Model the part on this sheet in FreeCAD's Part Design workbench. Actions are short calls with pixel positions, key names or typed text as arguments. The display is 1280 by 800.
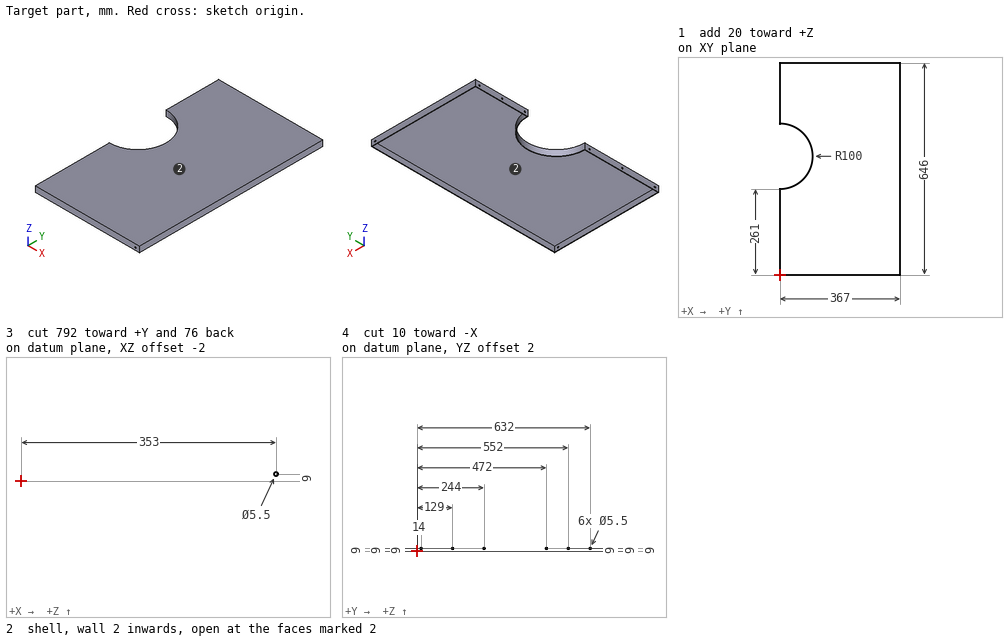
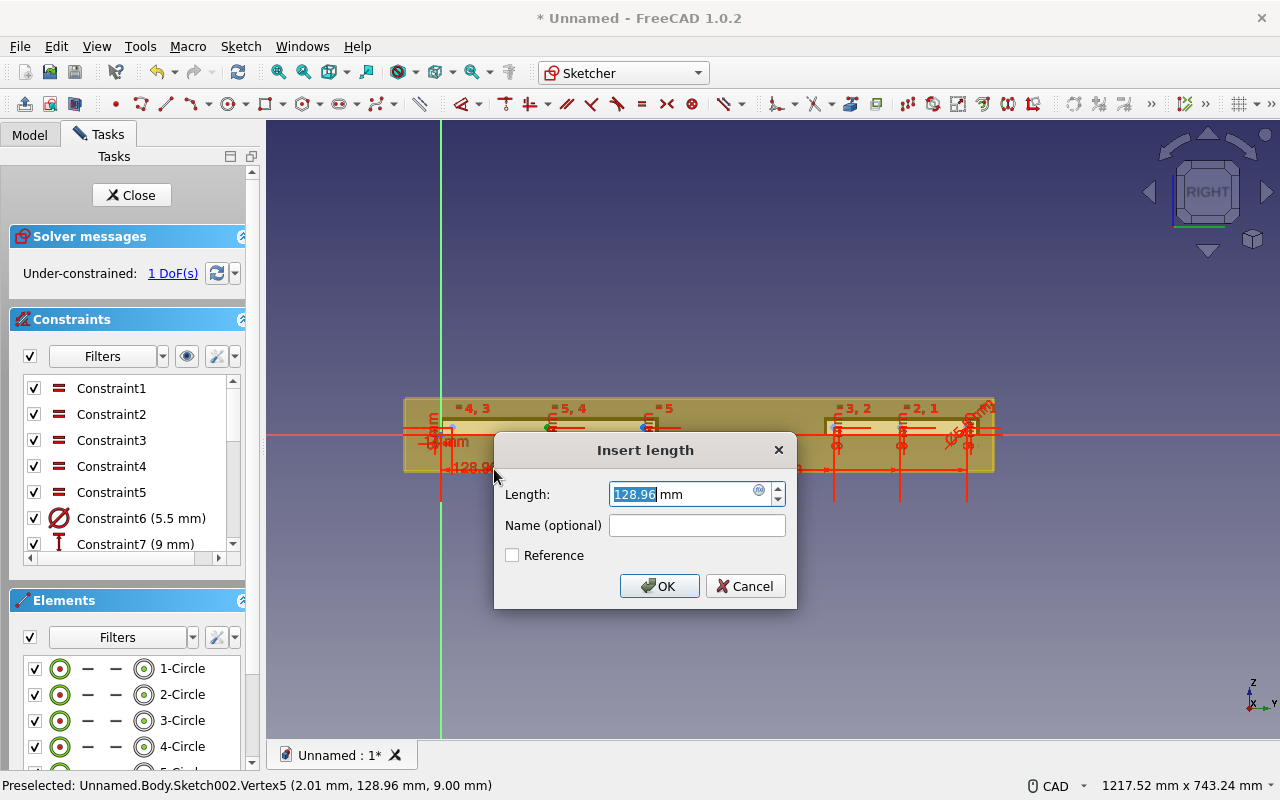
text(129)
key(Return)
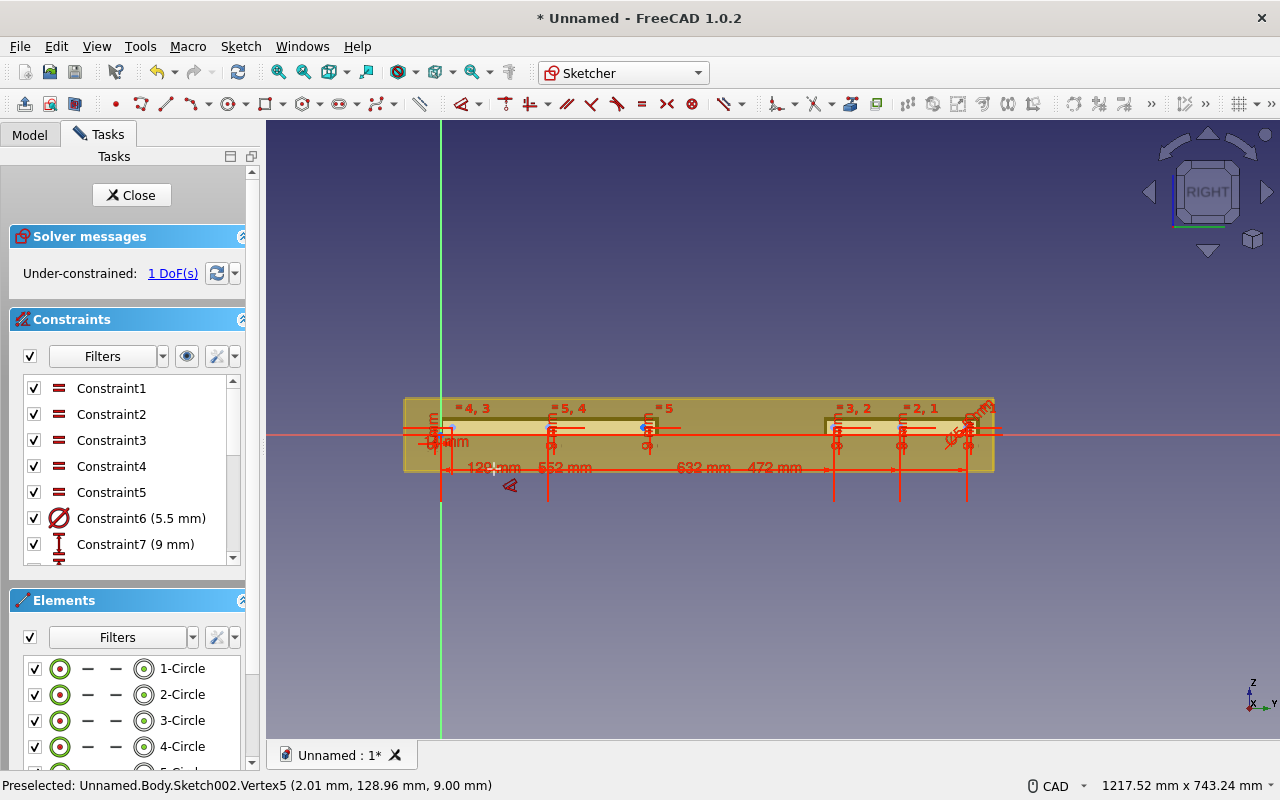
click(644, 428)
click(542, 394)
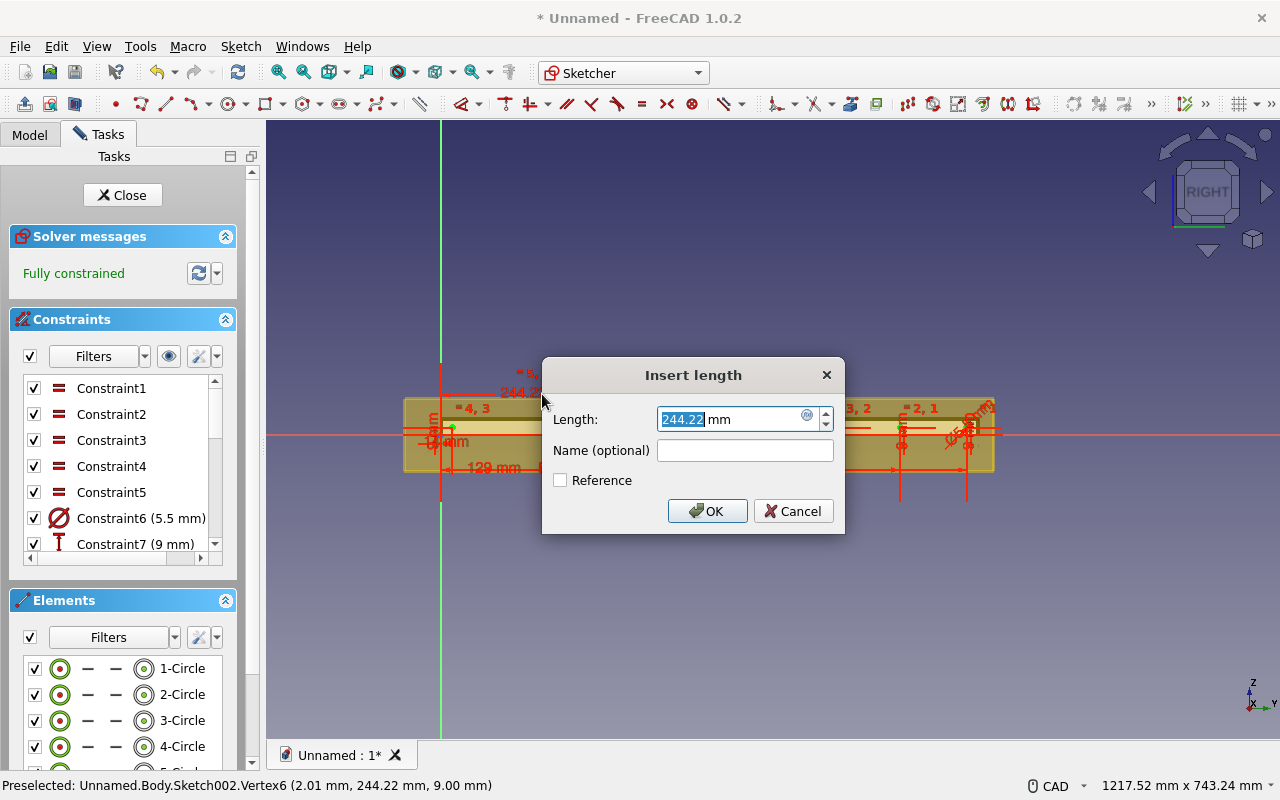
text(244)
key(Return)
key(Escape)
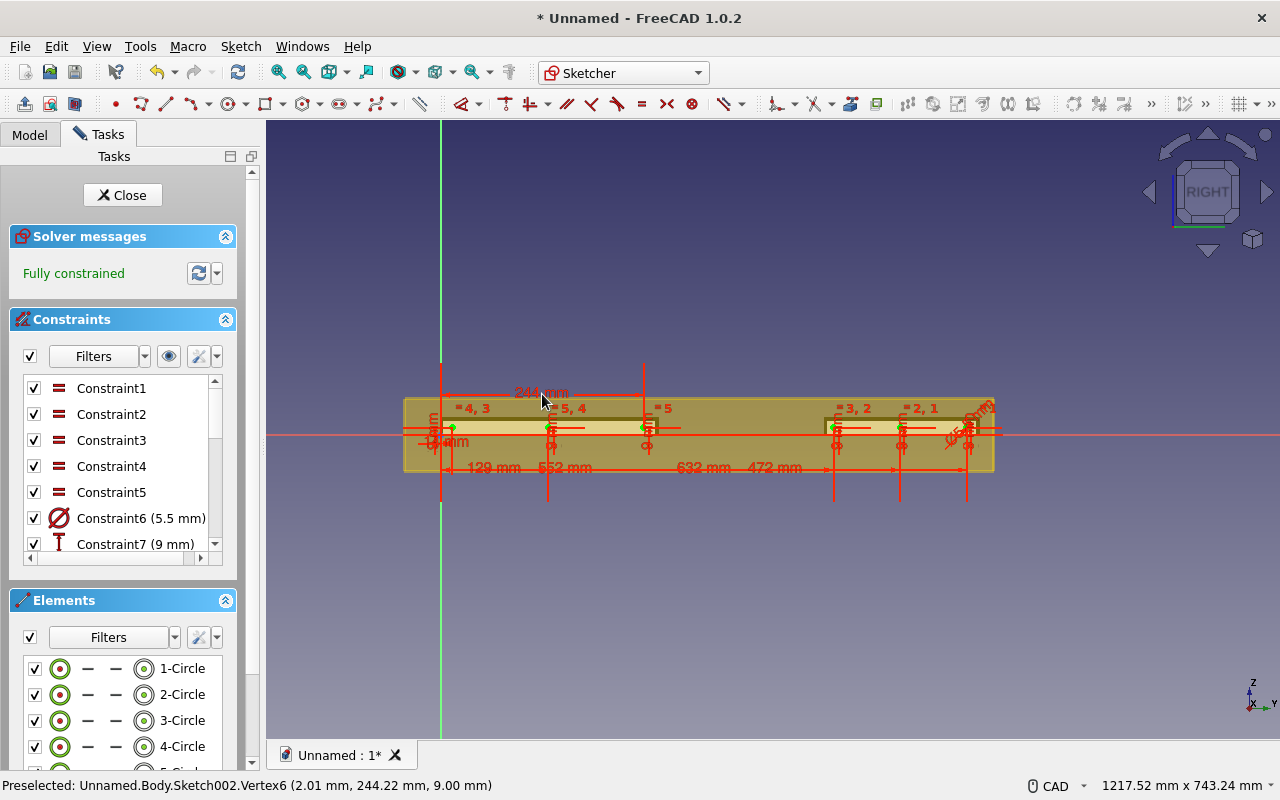
click(123, 195)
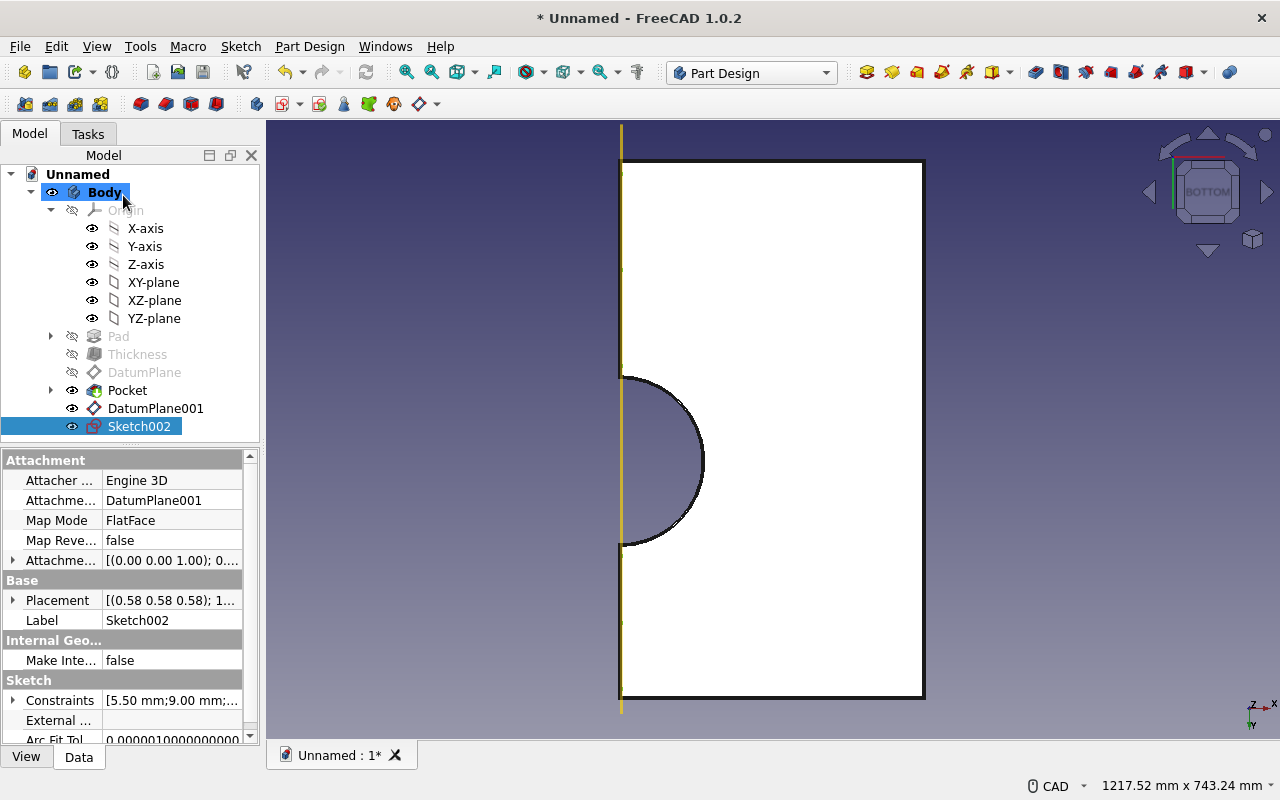
click(1036, 72)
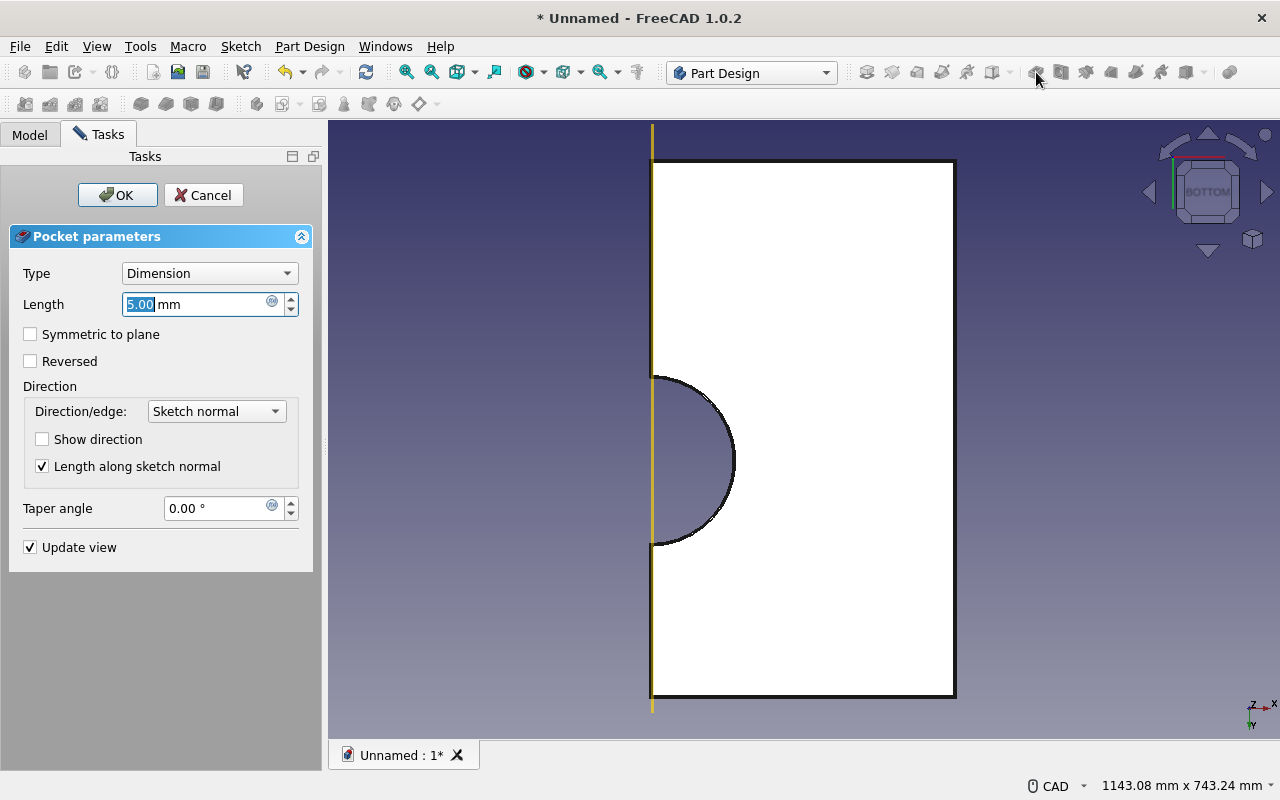
text(10)
key(Tab)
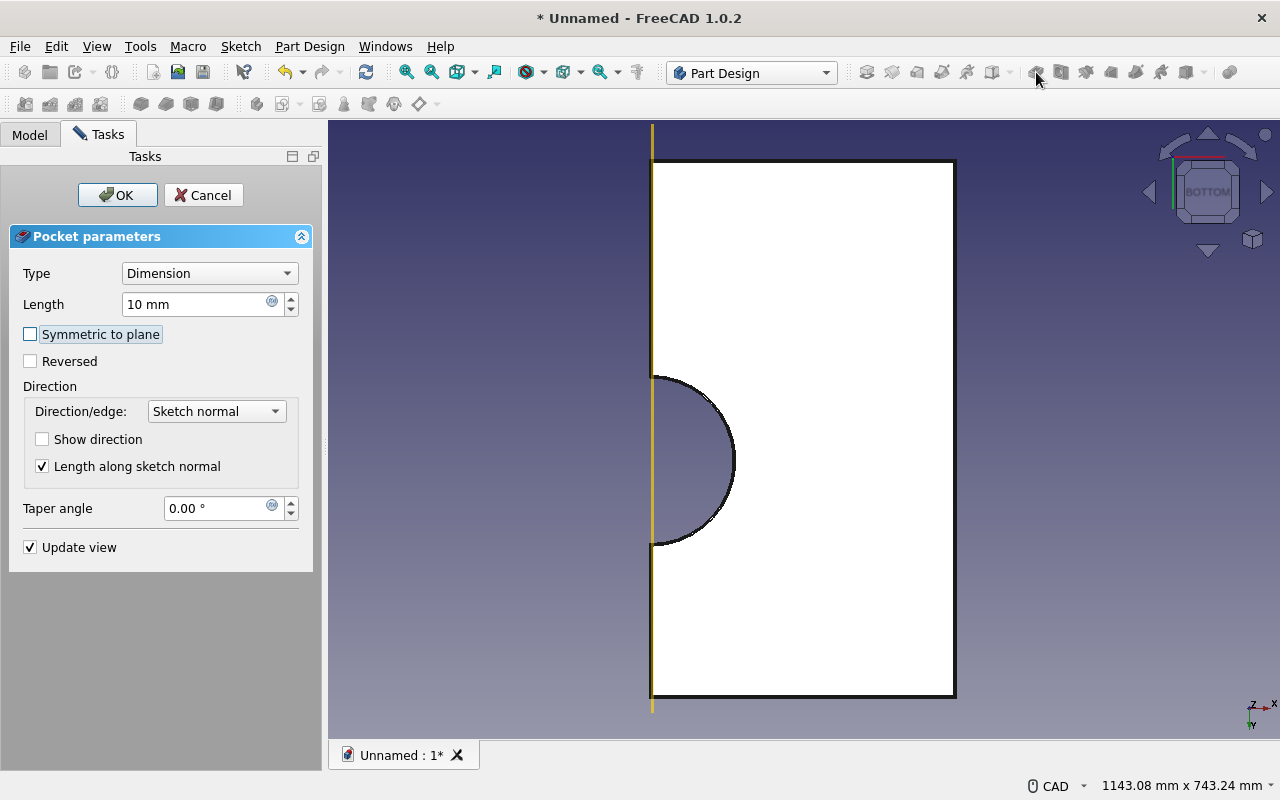
click(118, 195)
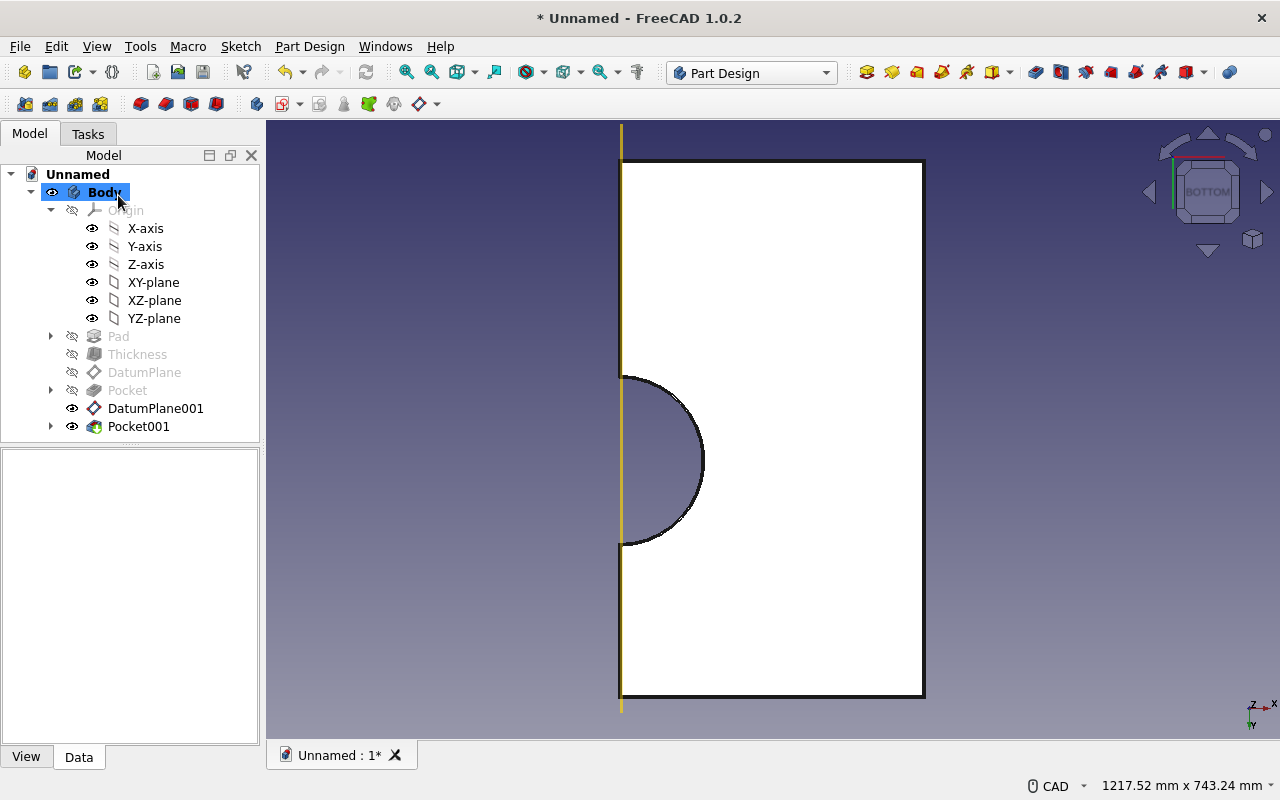
click(117, 408)
key(space)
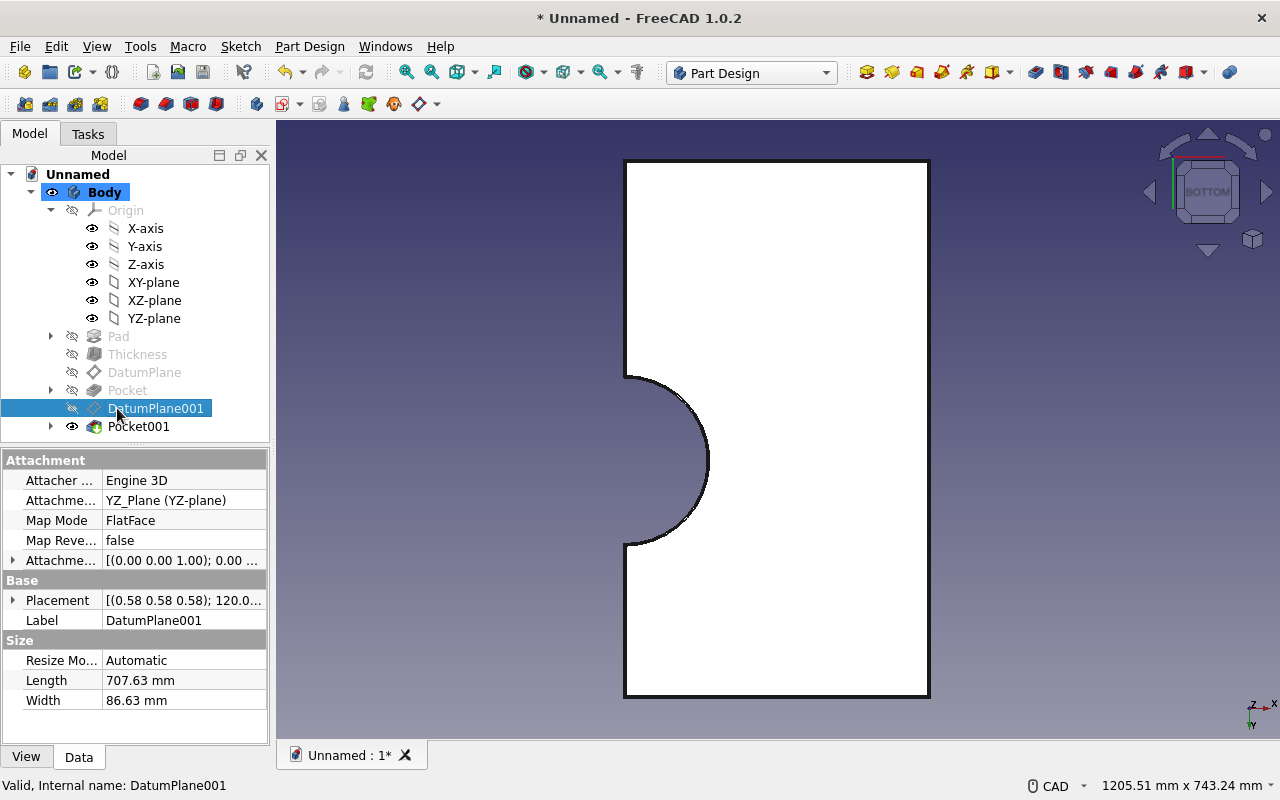
key(0)